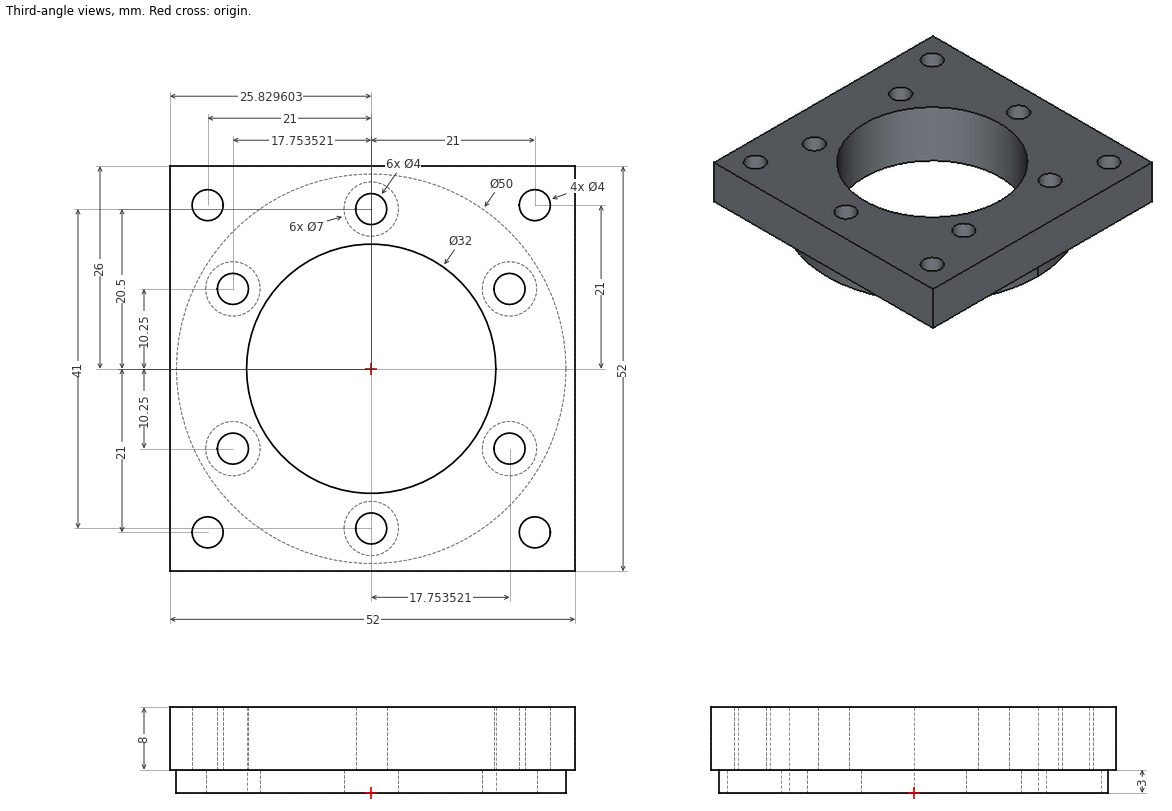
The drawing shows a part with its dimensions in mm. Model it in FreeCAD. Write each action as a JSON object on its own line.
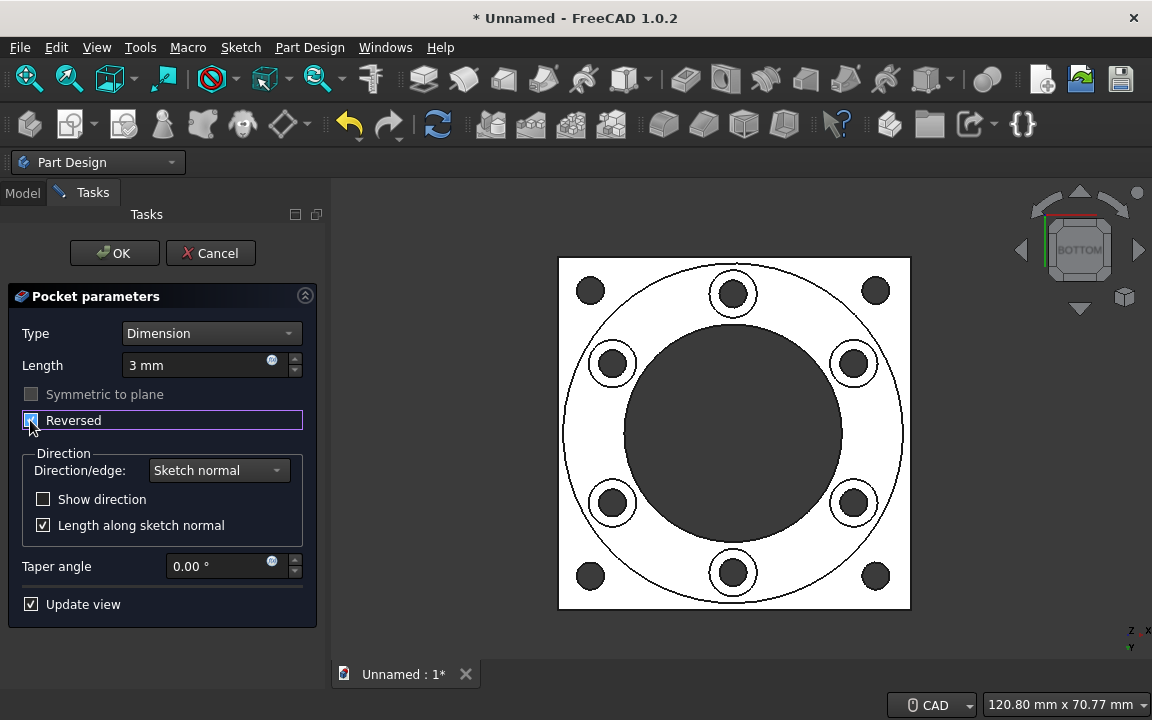
{"action": "left_click", "coordinate": [115, 253]}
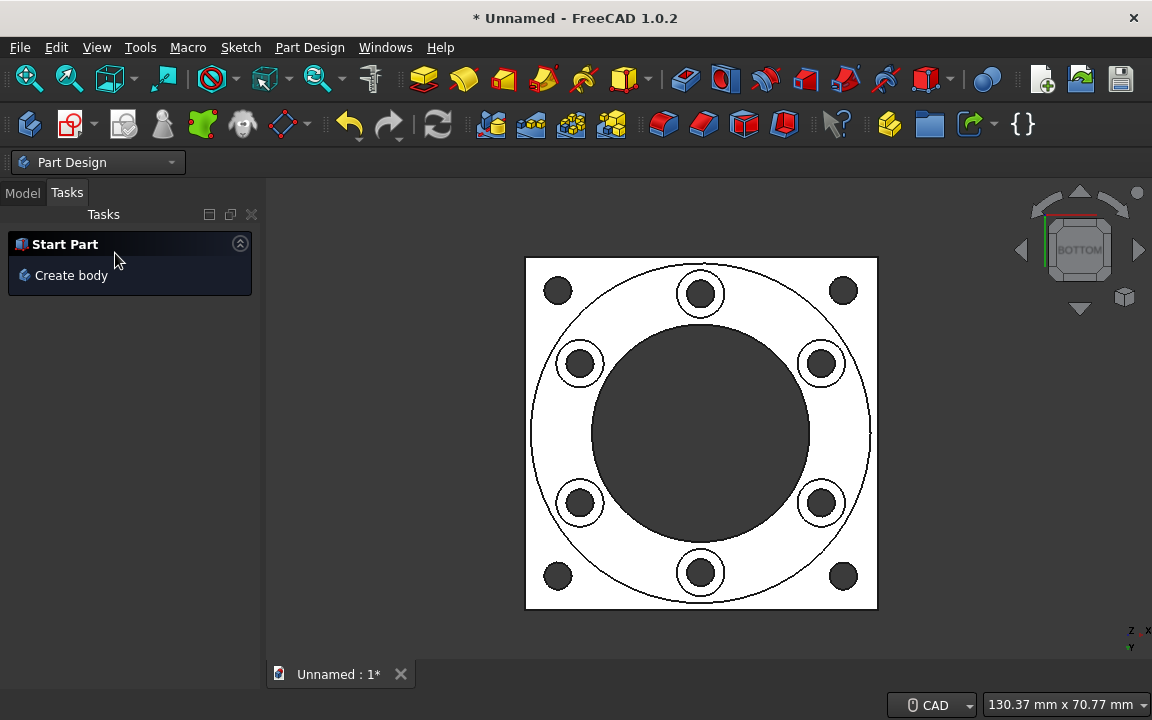
{"action": "key", "text": "0"}